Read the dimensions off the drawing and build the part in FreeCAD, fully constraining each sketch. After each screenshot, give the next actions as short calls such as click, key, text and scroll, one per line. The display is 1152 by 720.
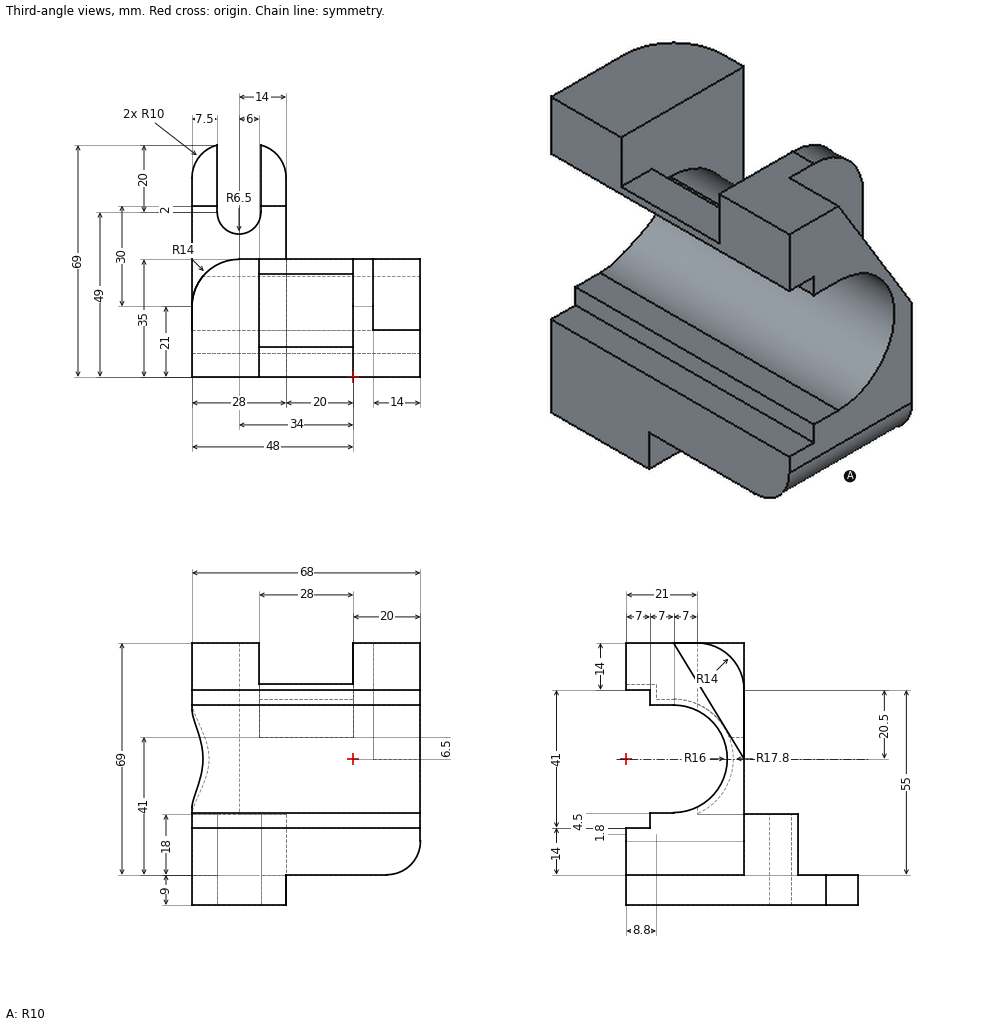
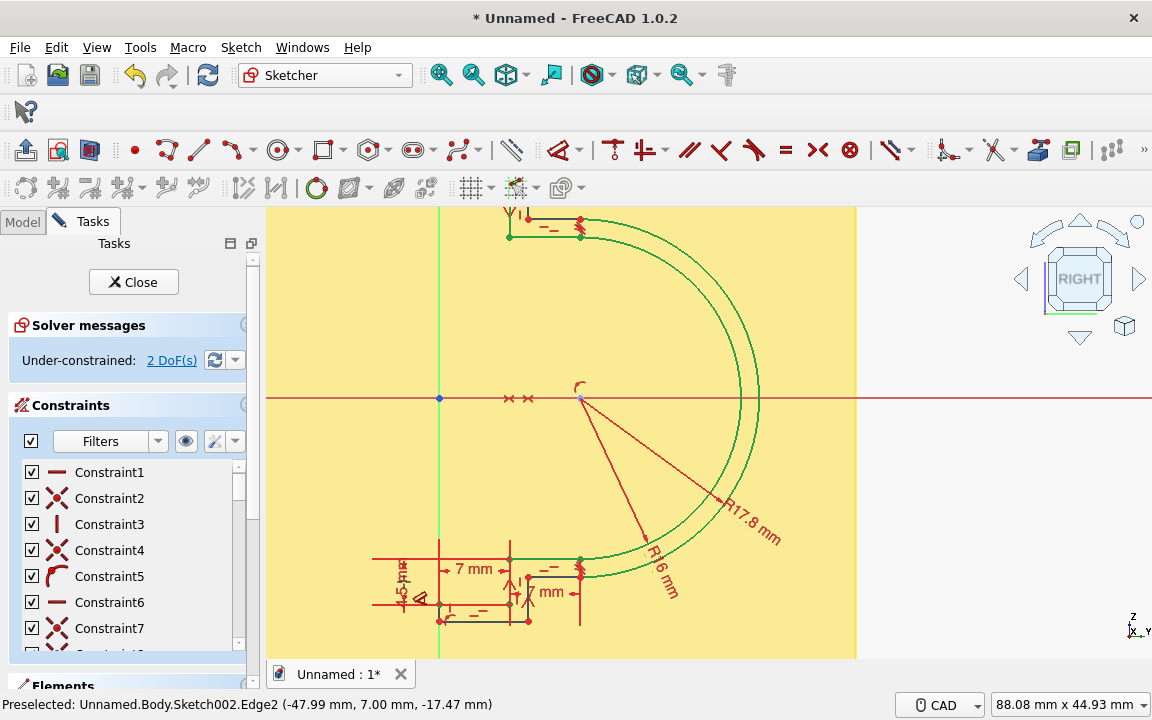
scroll(439, 613, up, 4)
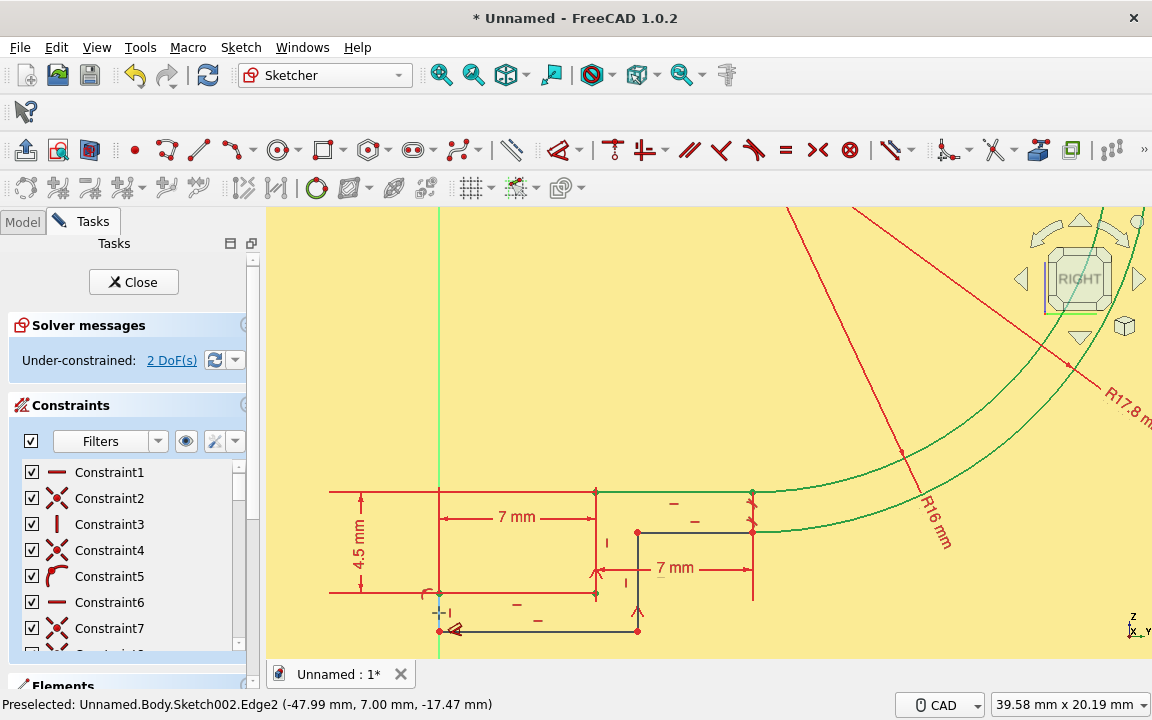
click(439, 612)
click(405, 612)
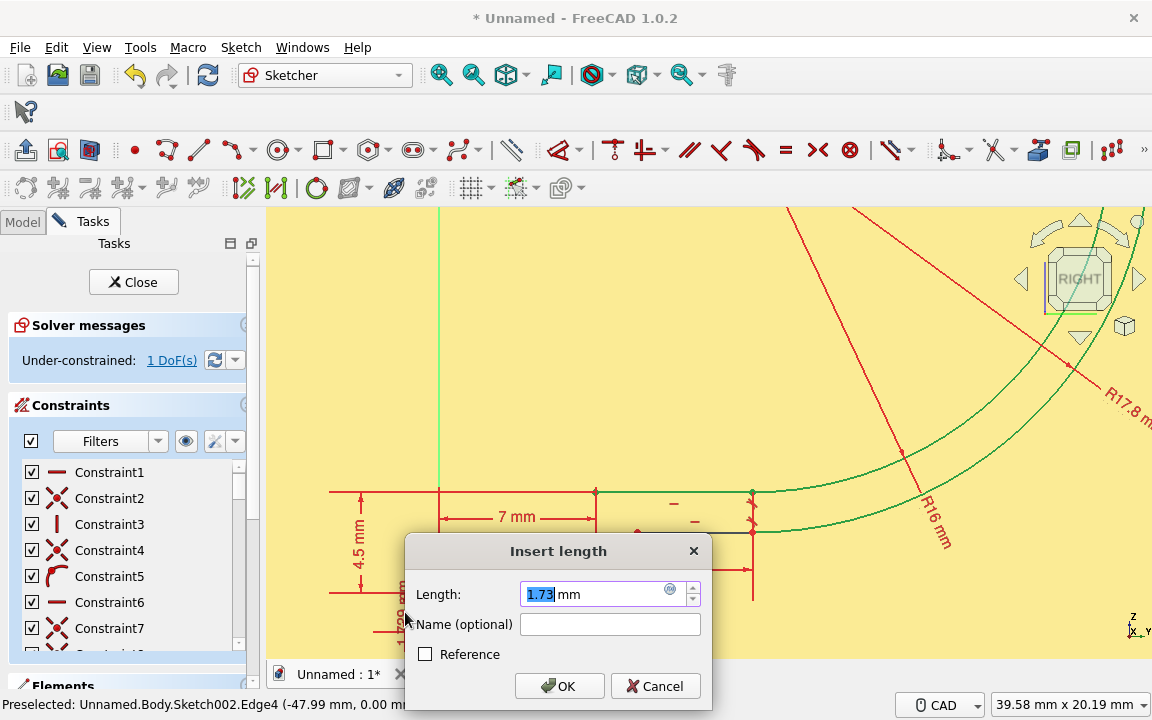
text(1.8)
key(Return)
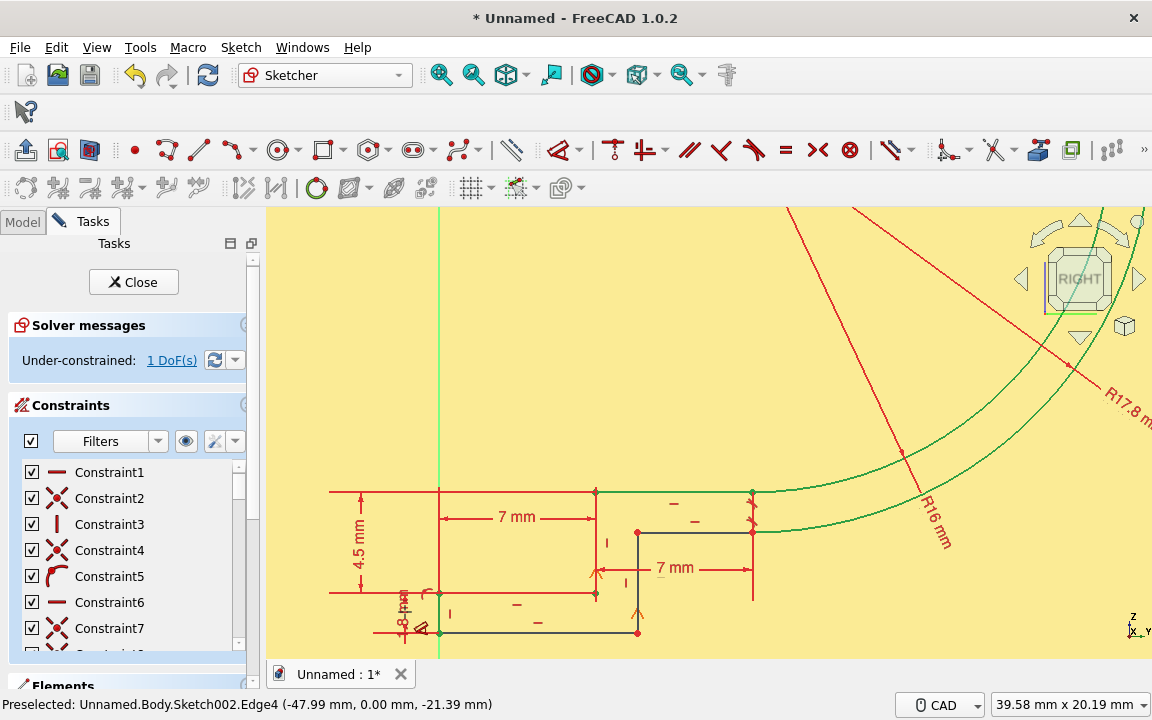
scroll(574, 562, down, 6)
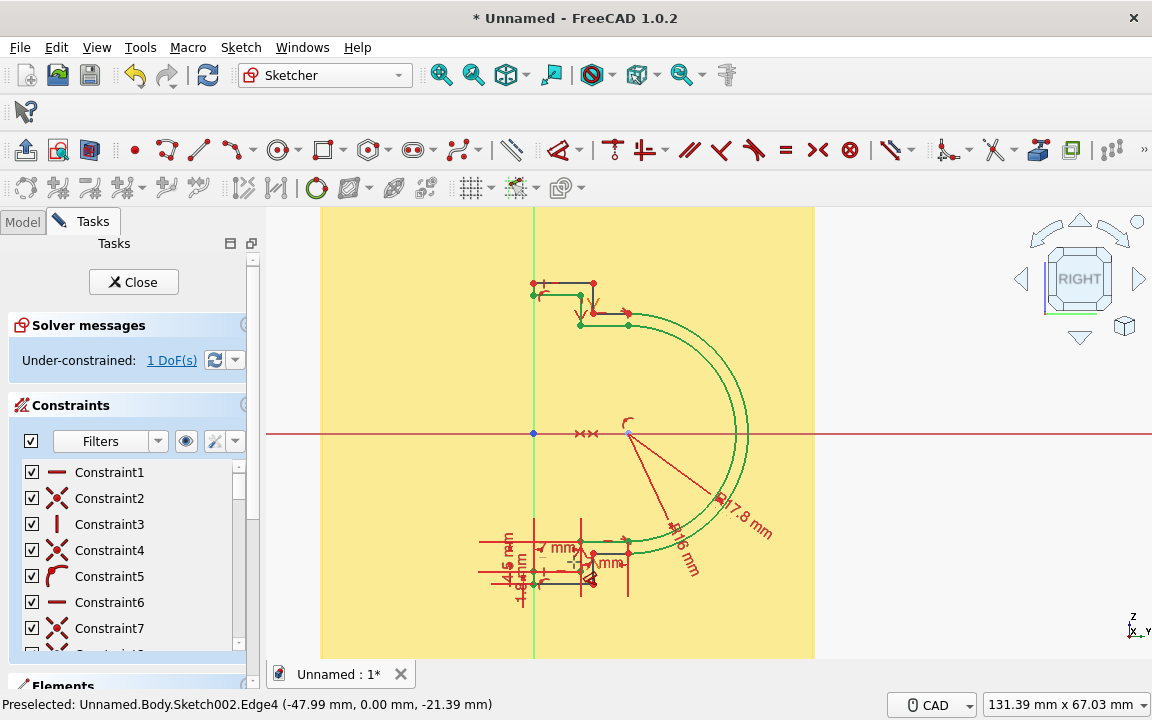
click(552, 584)
click(564, 618)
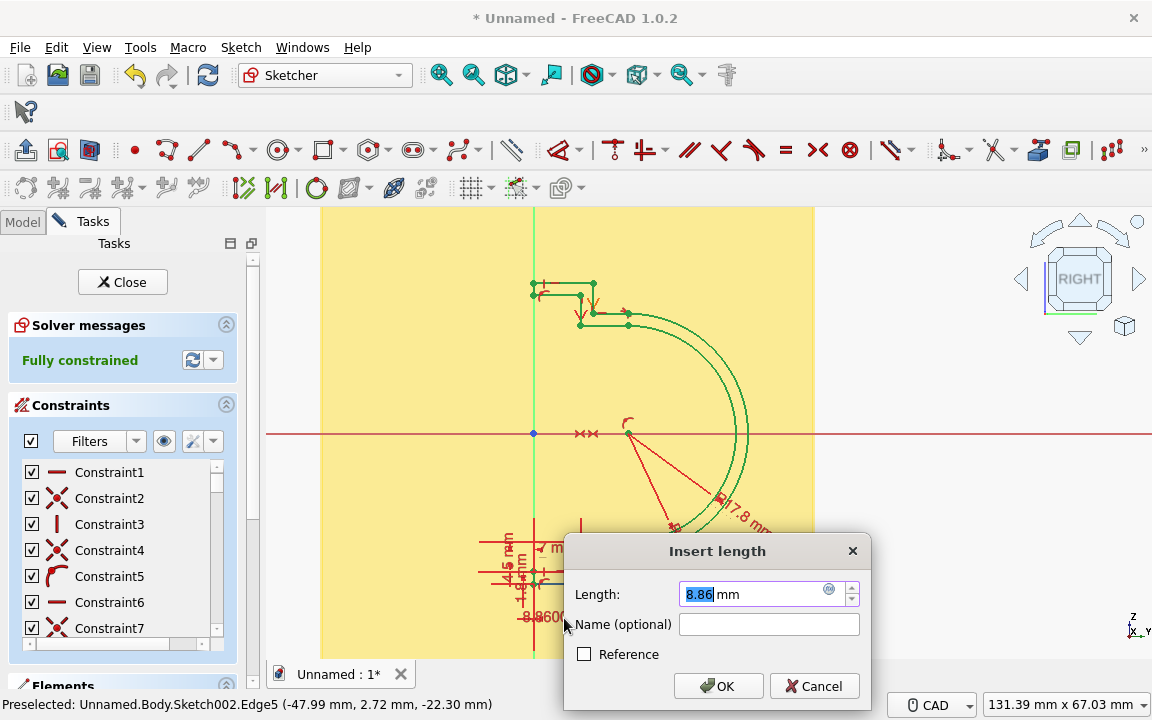
text(8.8)
key(Return)
key(Escape)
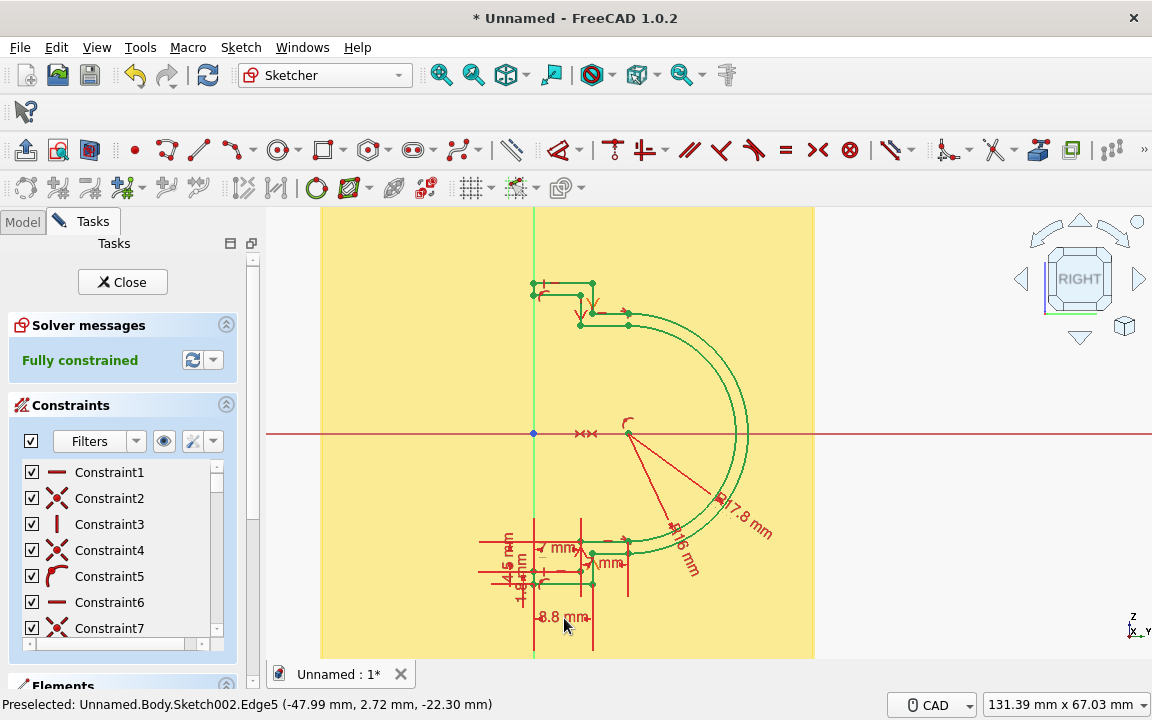
click(123, 282)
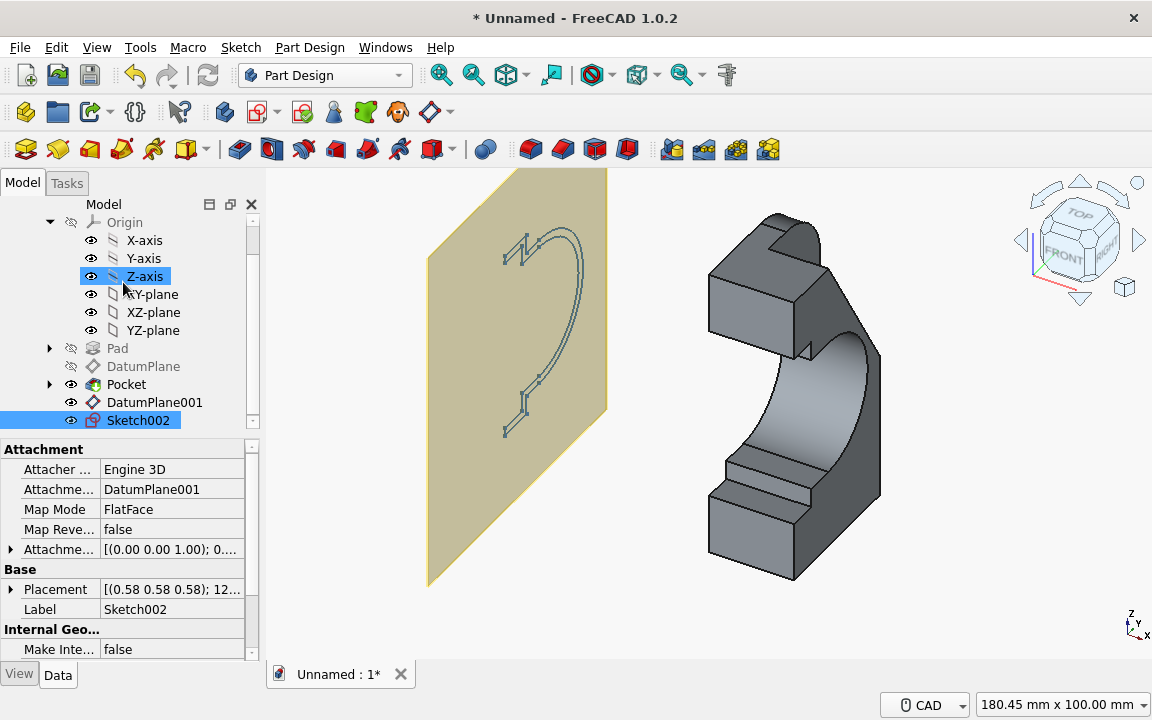
click(26, 150)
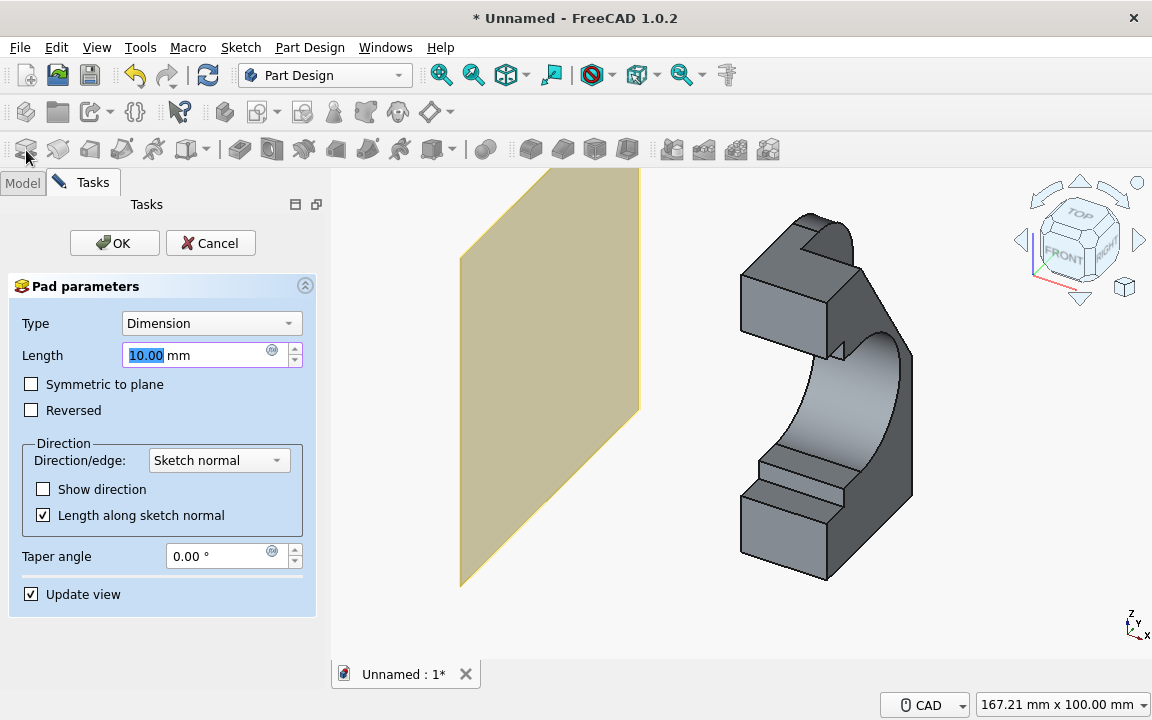
text(68)
key(Tab)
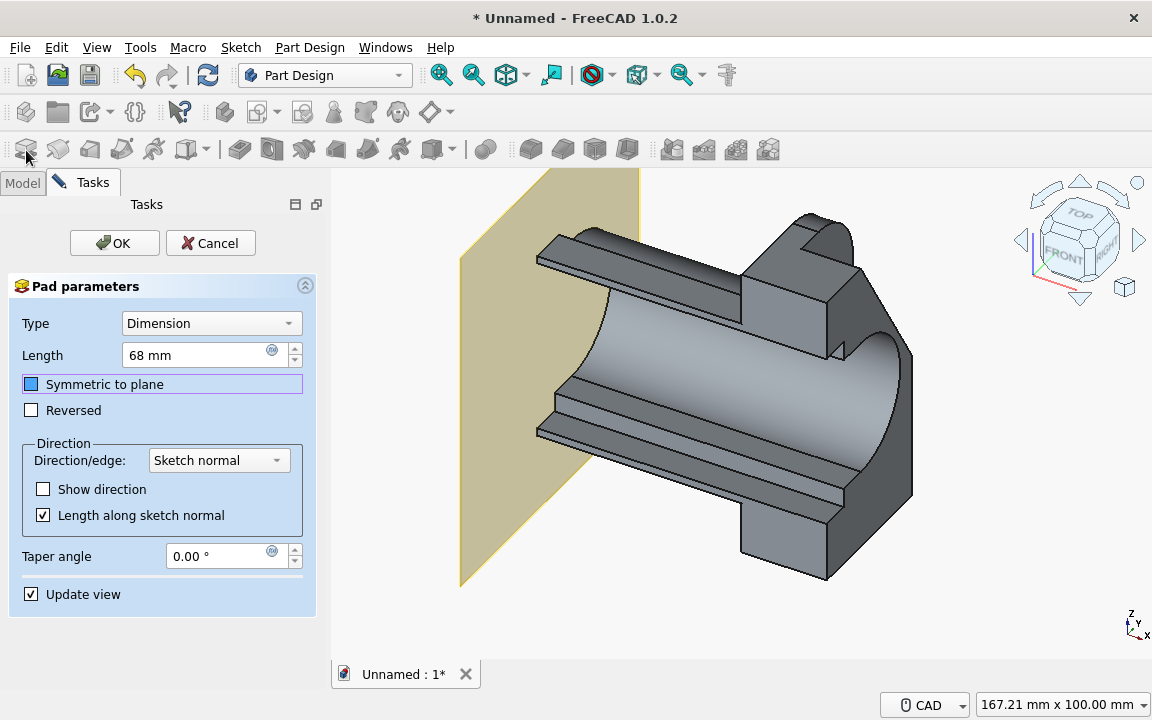
click(115, 243)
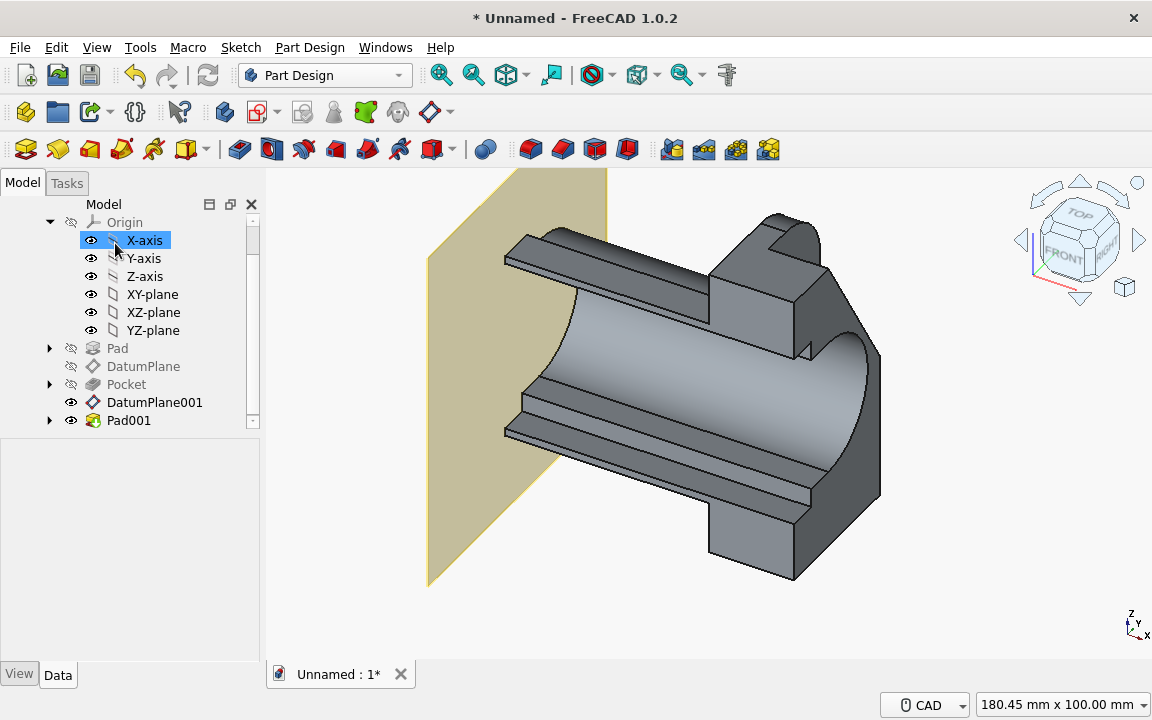
click(116, 402)
key(space)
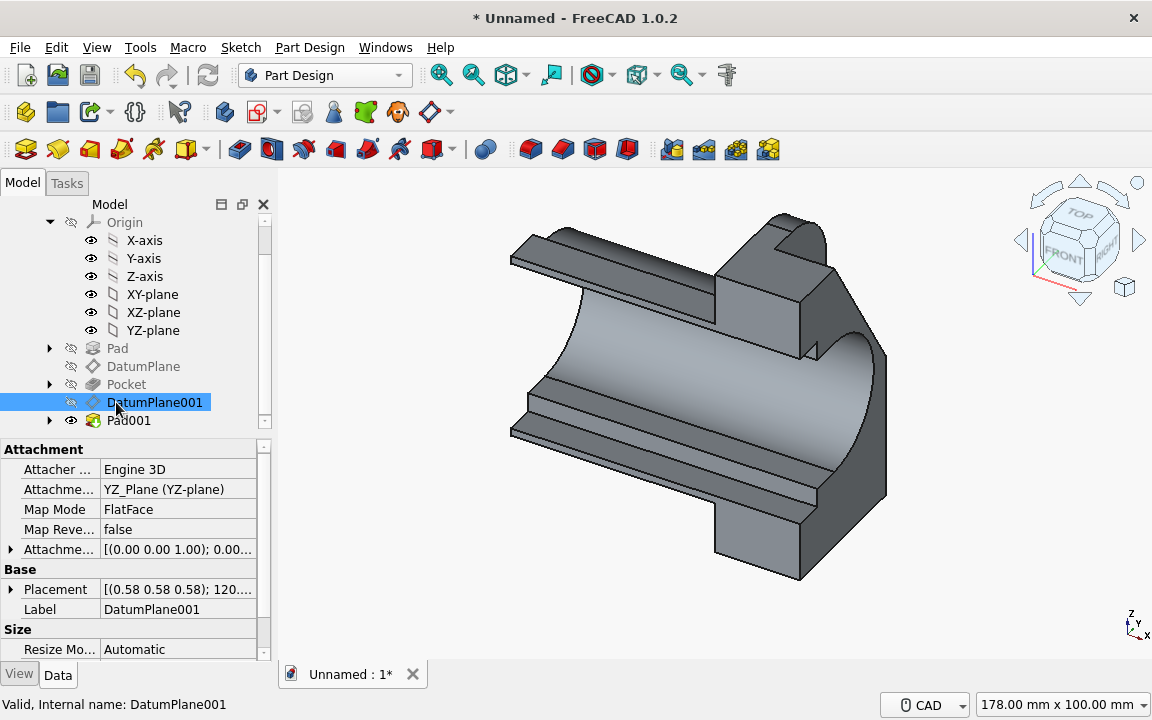
key(v)
key(f)